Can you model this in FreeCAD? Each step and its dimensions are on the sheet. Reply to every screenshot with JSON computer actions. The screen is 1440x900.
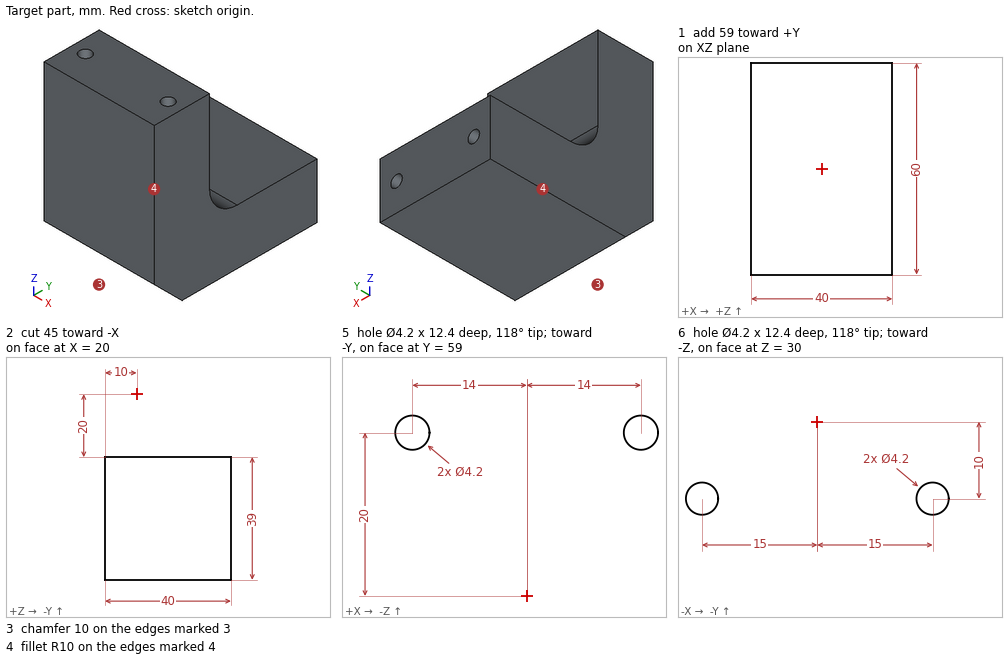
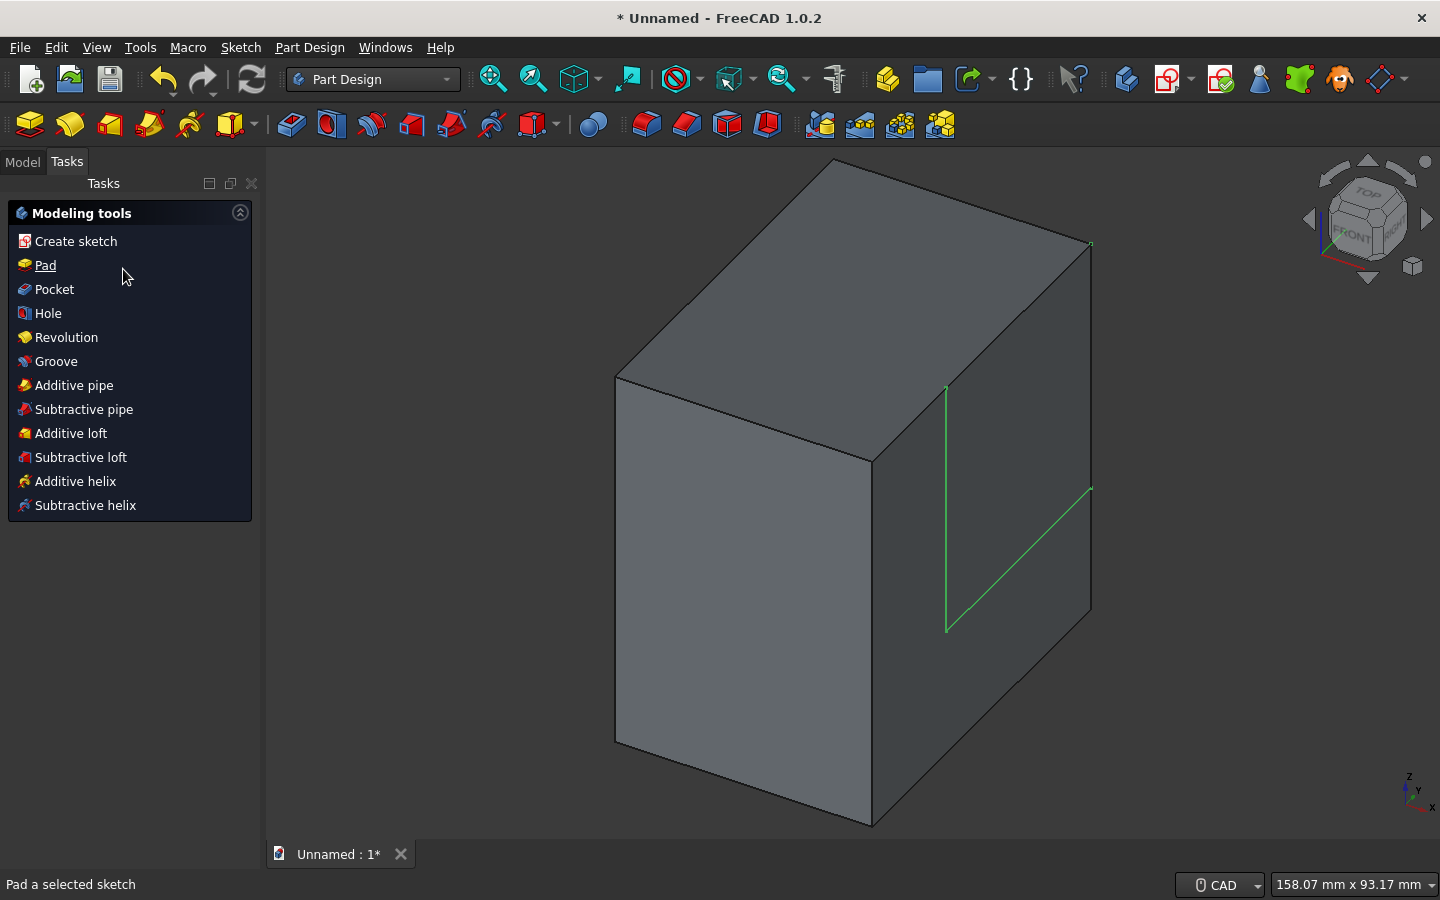
{"action": "left_click", "coordinate": [292, 124]}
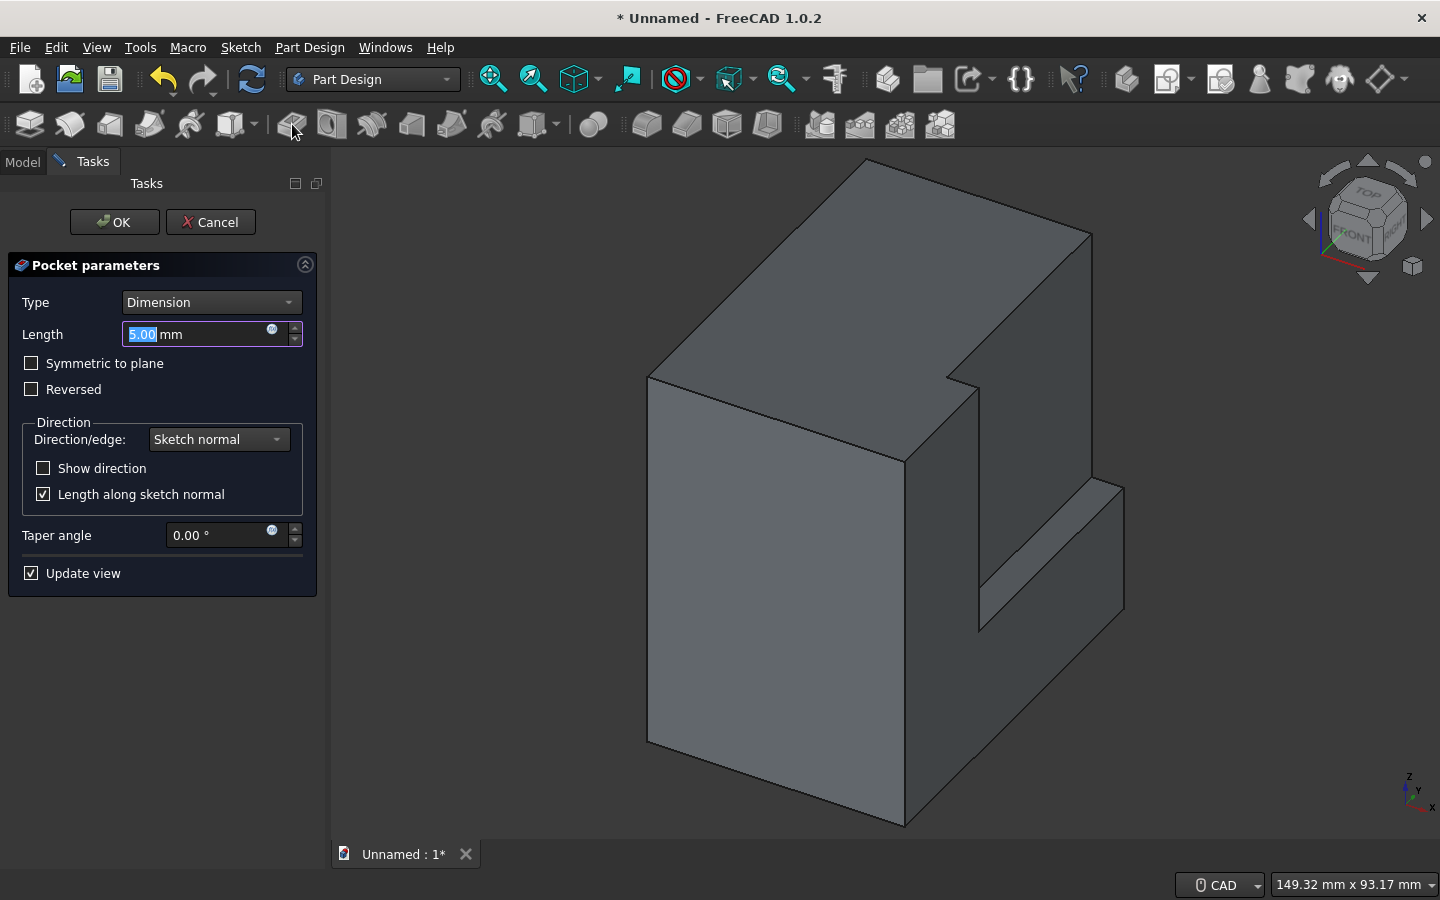
{"action": "type", "text": "45"}
{"action": "key", "text": "Tab"}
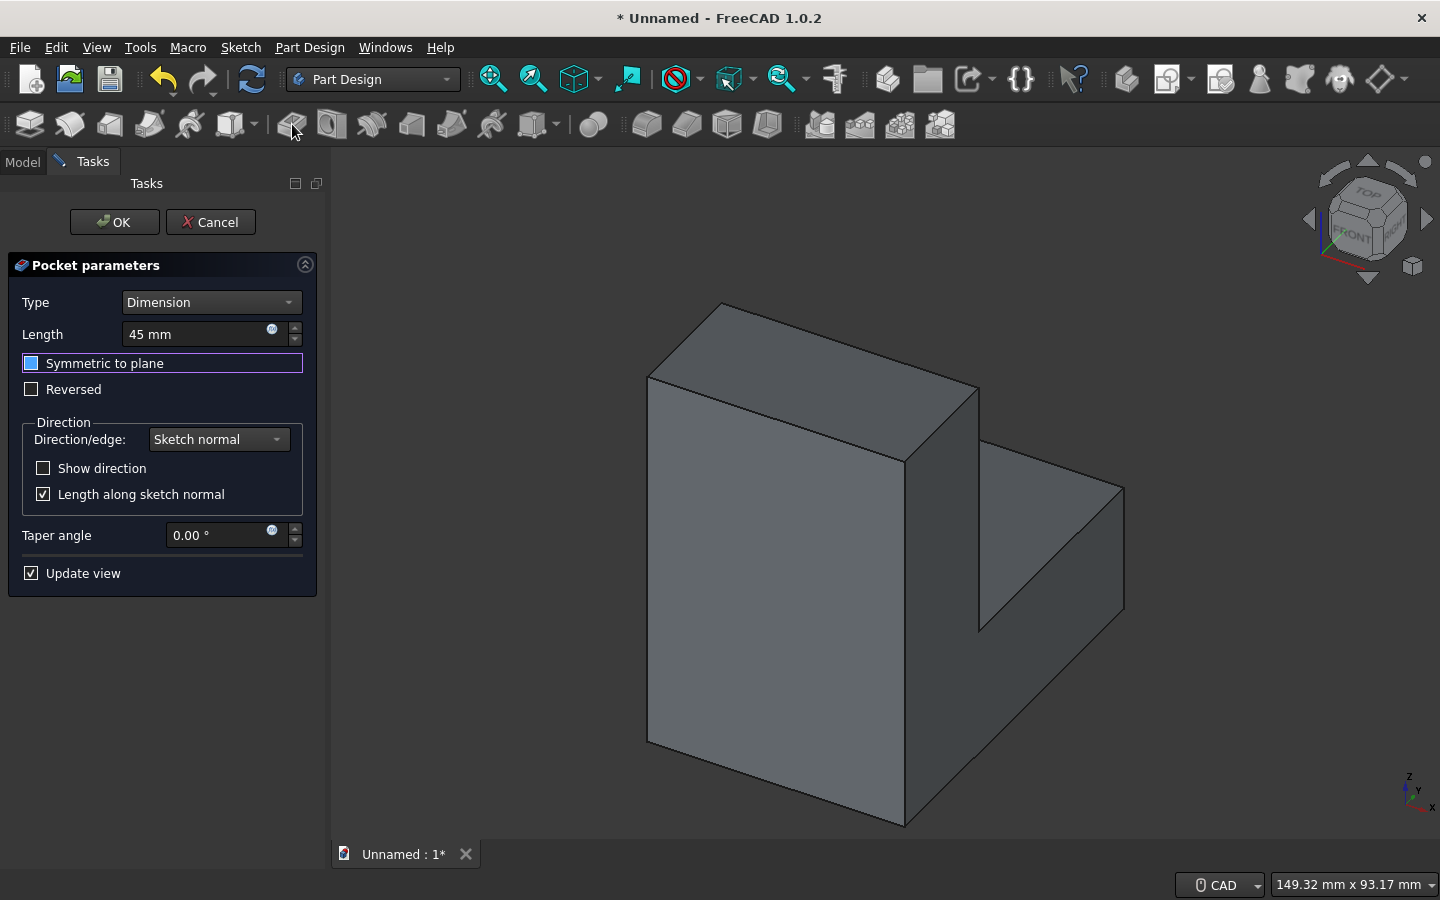
{"action": "left_click", "coordinate": [115, 222]}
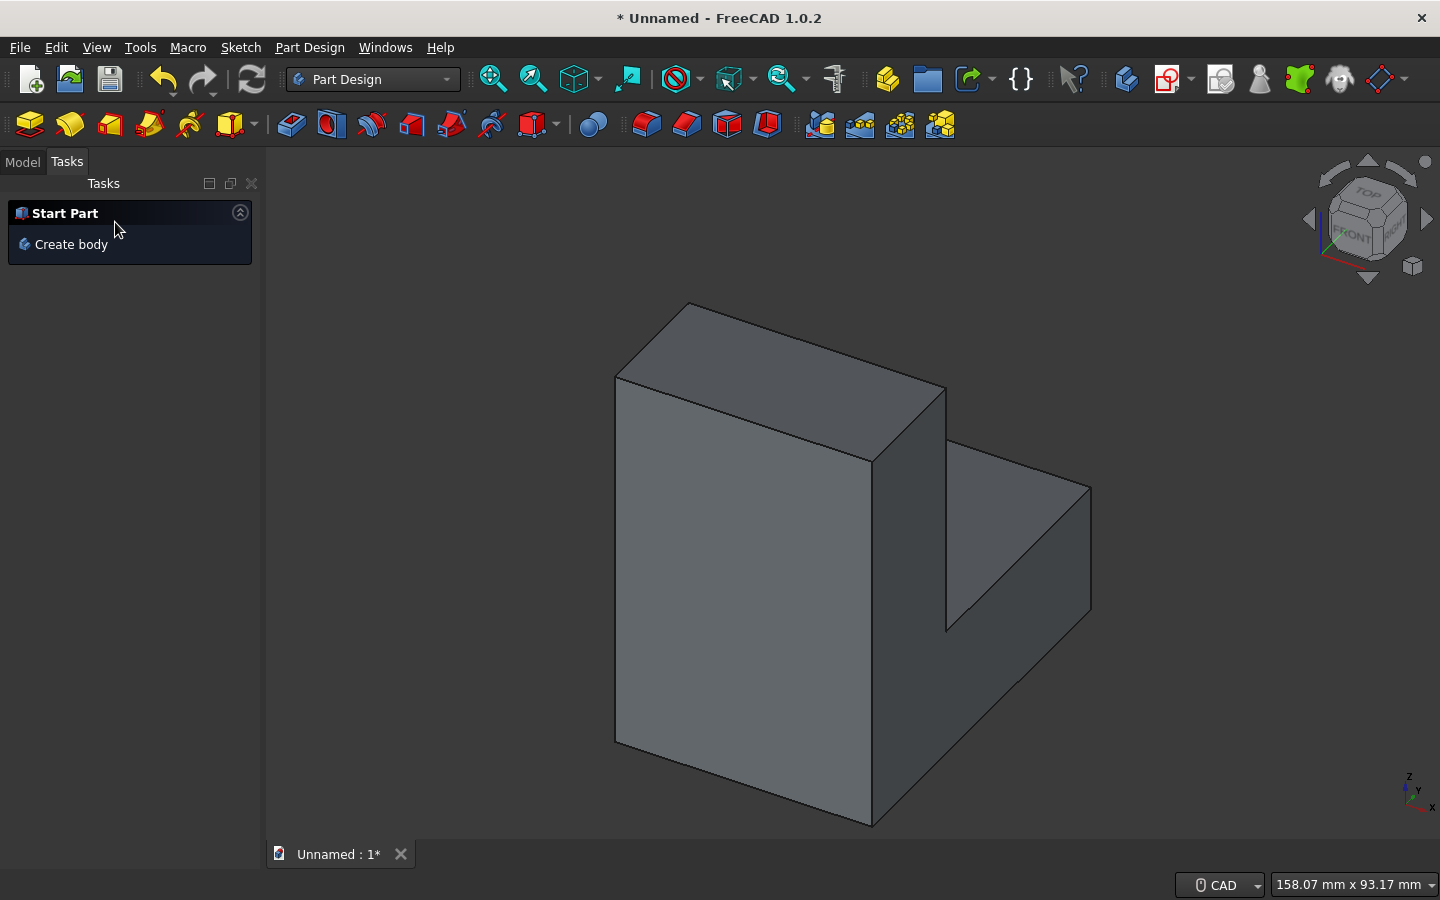
{"action": "key", "text": "0"}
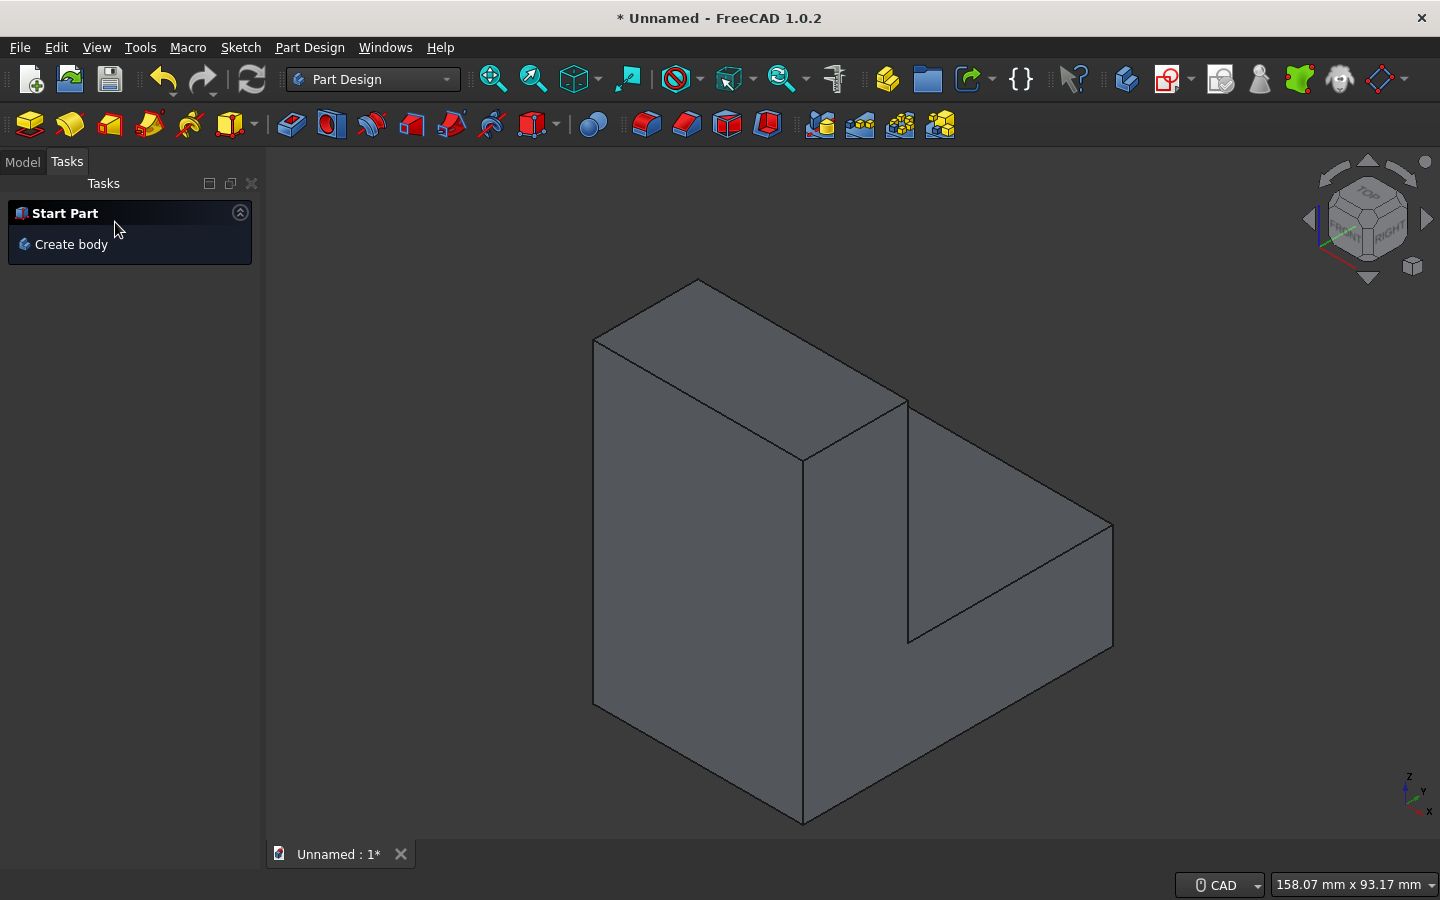
{"action": "key", "text": "2"}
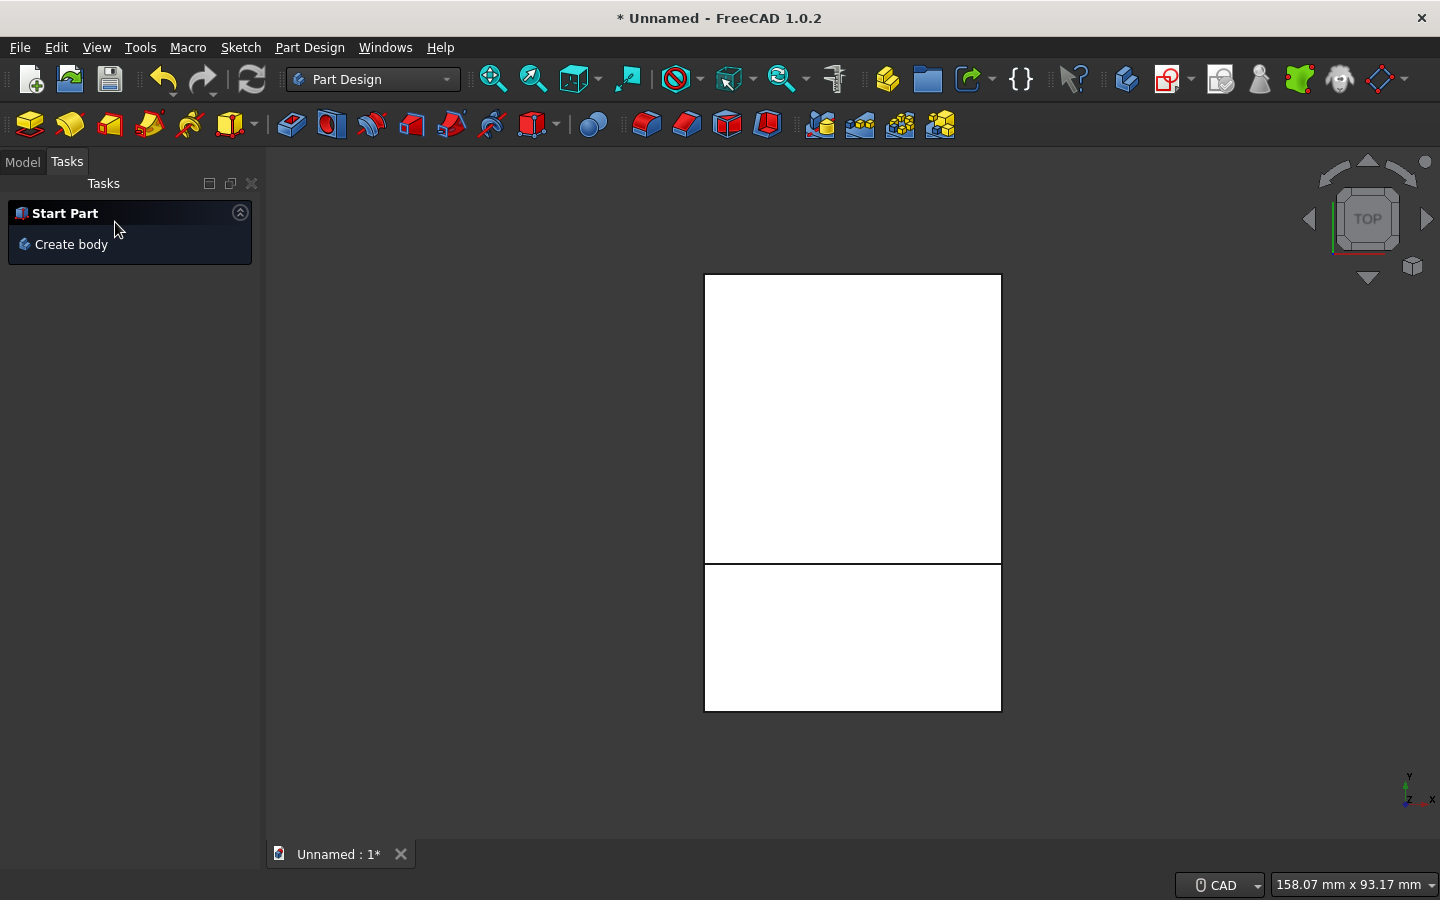
{"action": "key", "text": "1"}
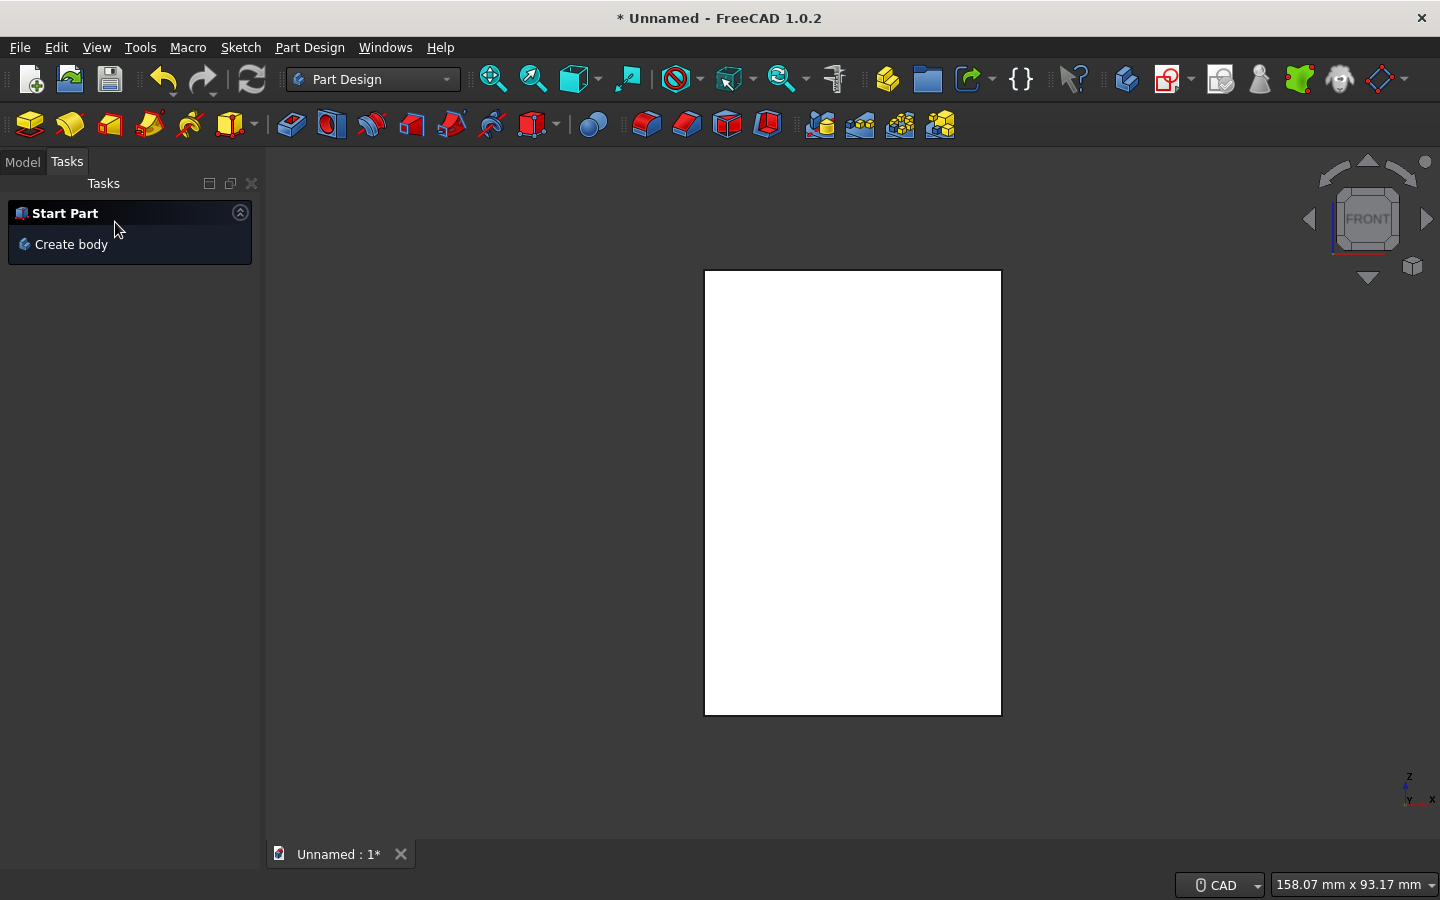
{"action": "key", "text": "3"}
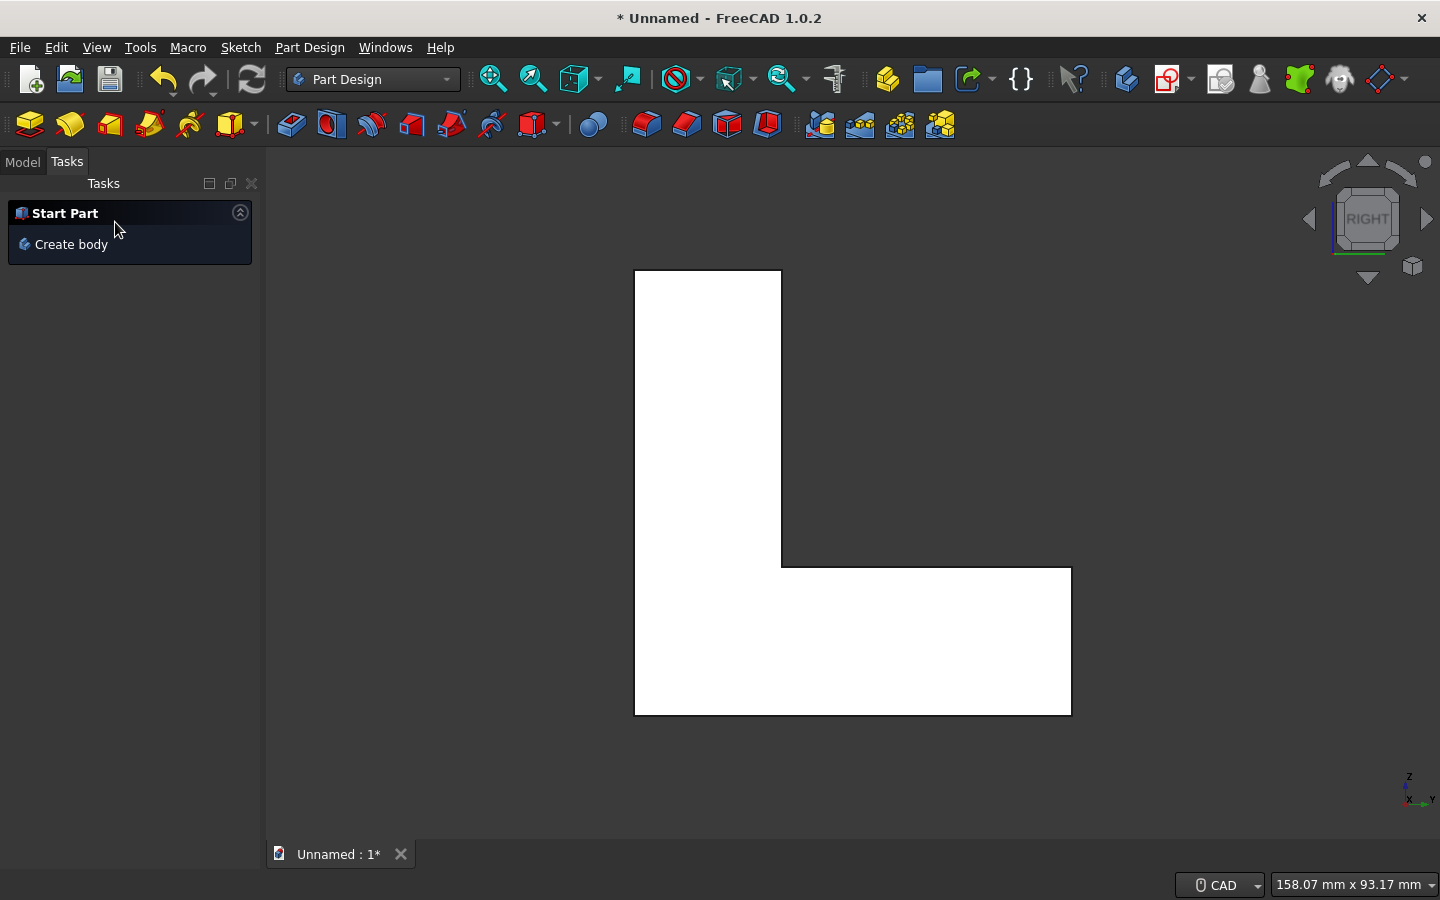
{"action": "key", "text": "5"}